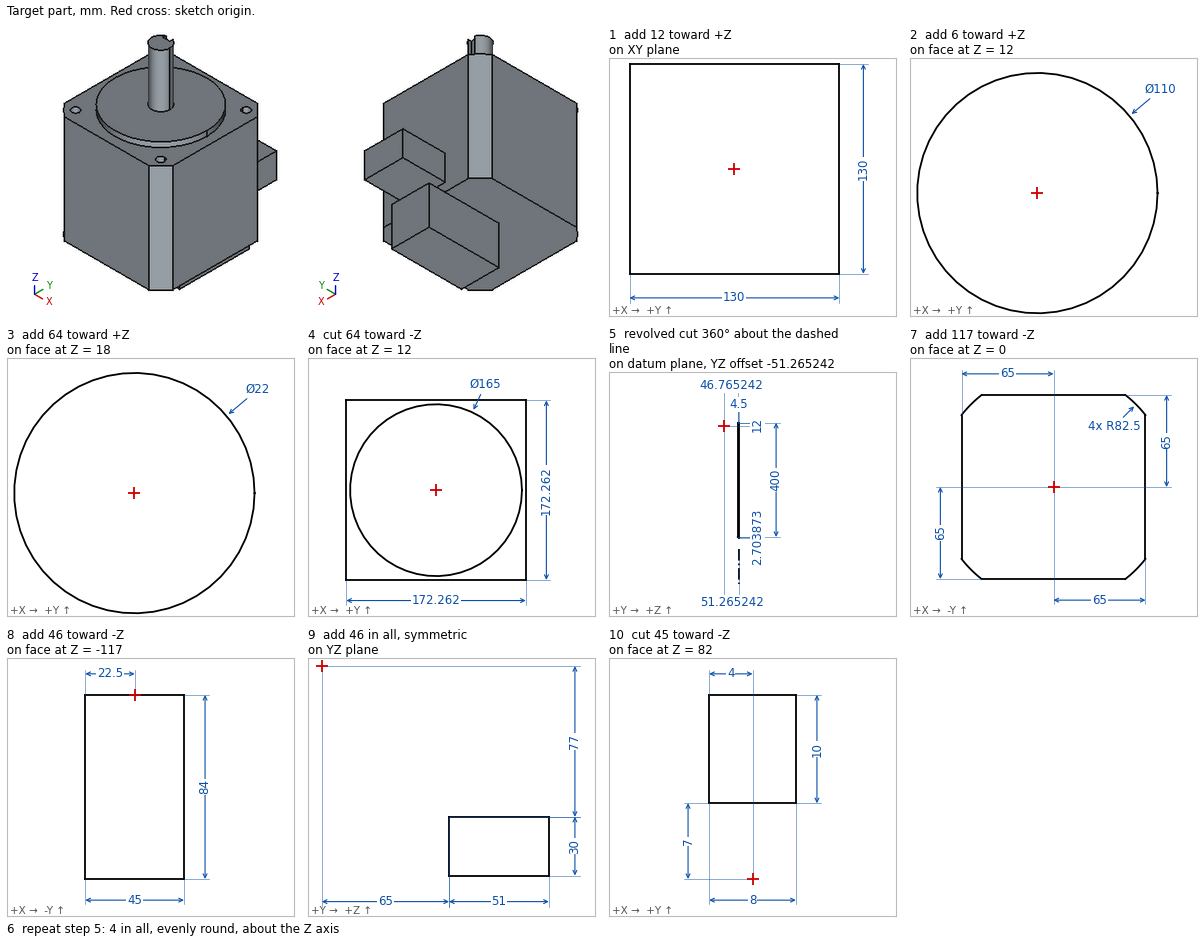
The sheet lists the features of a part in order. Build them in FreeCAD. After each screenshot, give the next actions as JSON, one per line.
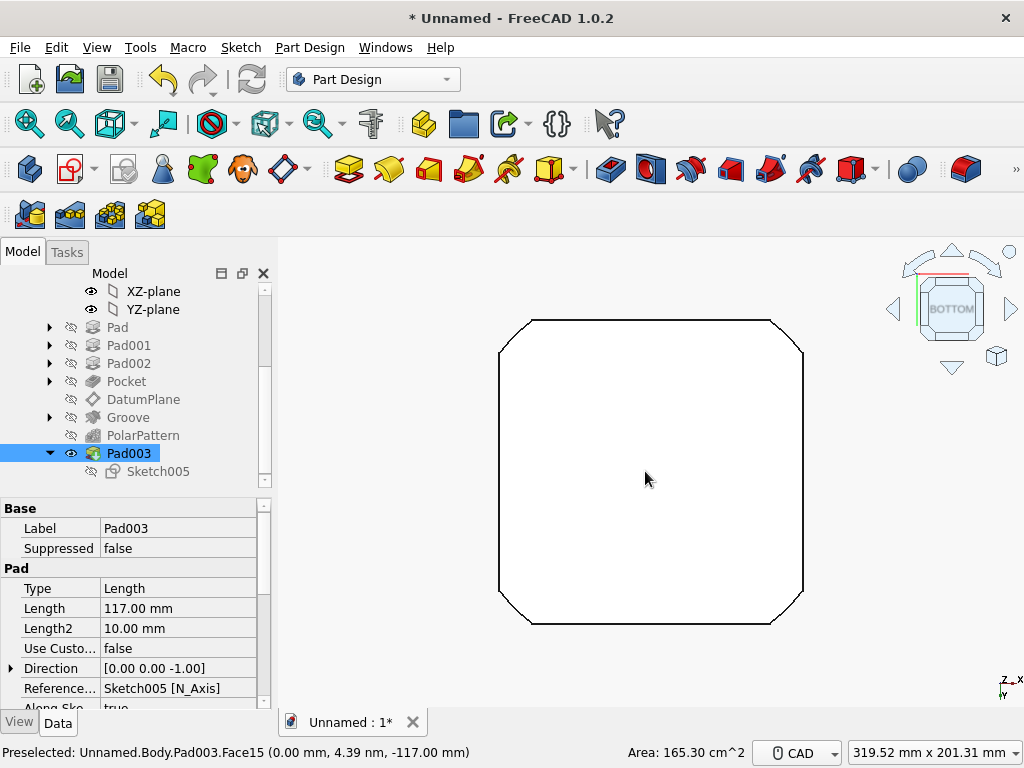
{"action": "left_click", "coordinate": [70, 170]}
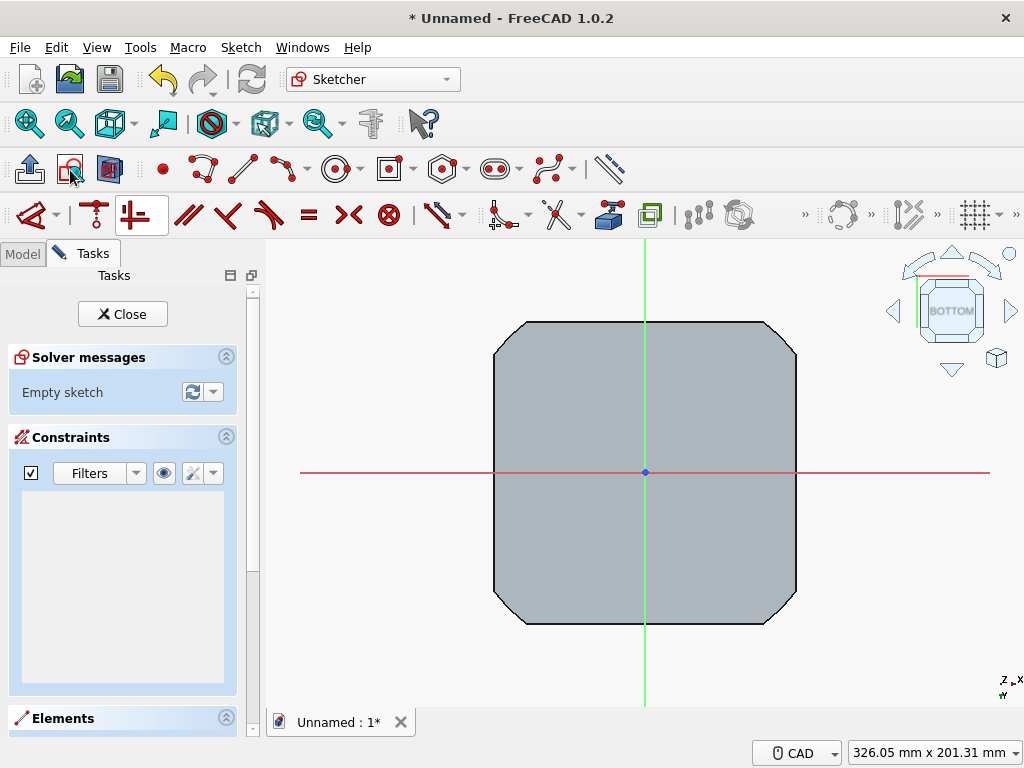
{"action": "scroll", "coordinate": [294, 267], "scroll_direction": "down", "scroll_amount": 1}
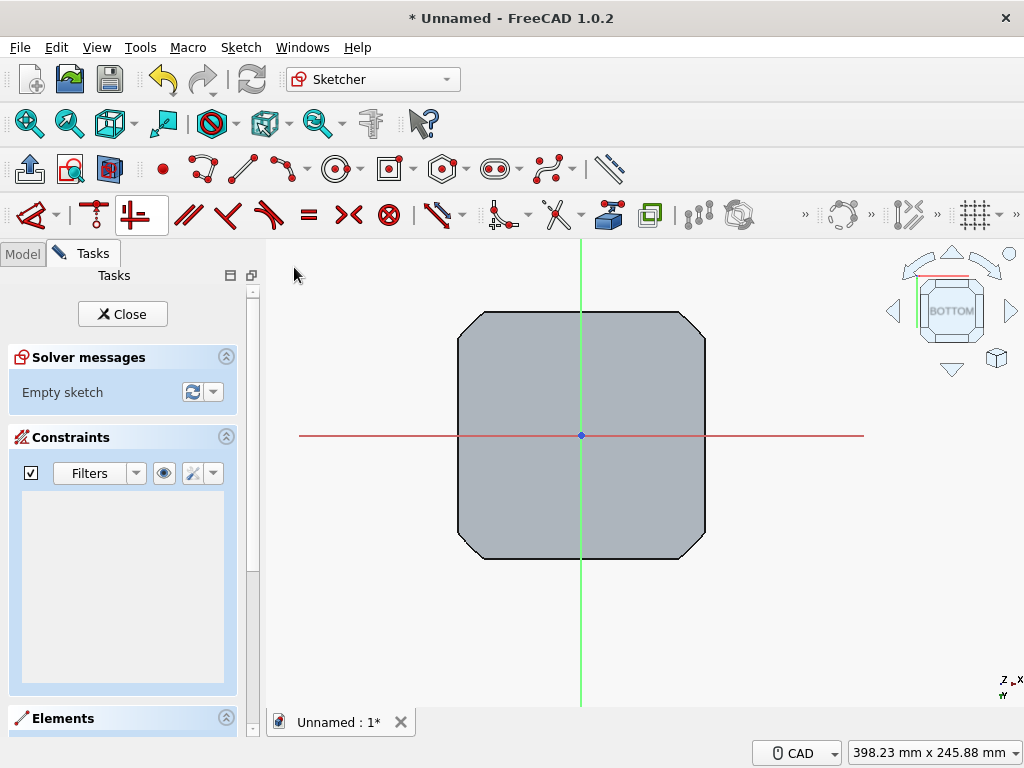
{"action": "scroll", "coordinate": [587, 567], "scroll_direction": "up", "scroll_amount": 3}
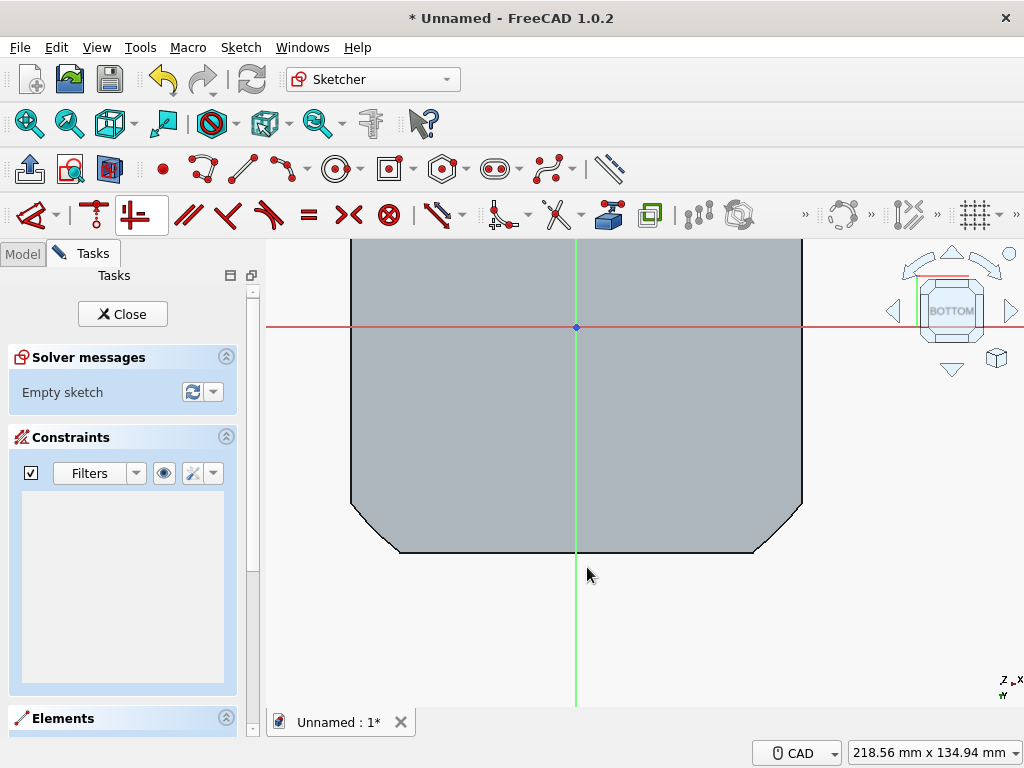
{"action": "key", "text": "g r"}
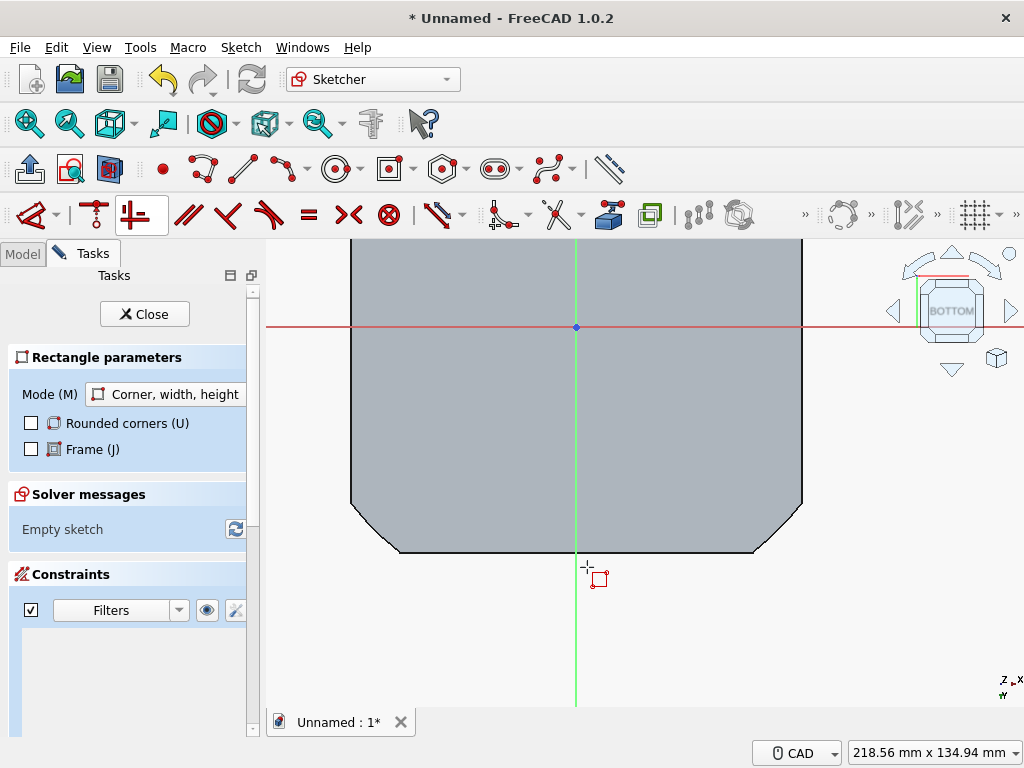
{"action": "left_click", "coordinate": [498, 327]}
{"action": "mouse_move", "coordinate": [654, 618]}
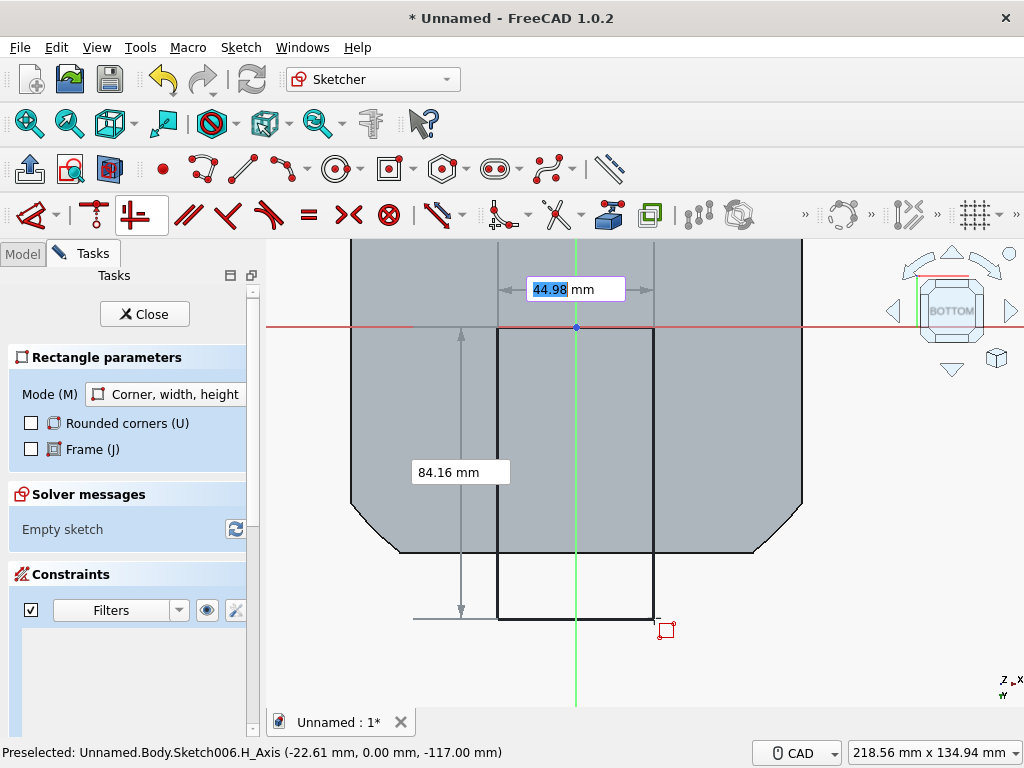
{"action": "type", "text": "45"}
{"action": "key", "text": "Tab"}
{"action": "type", "text": "84"}
{"action": "key", "text": "Return"}
{"action": "key", "text": "Escape"}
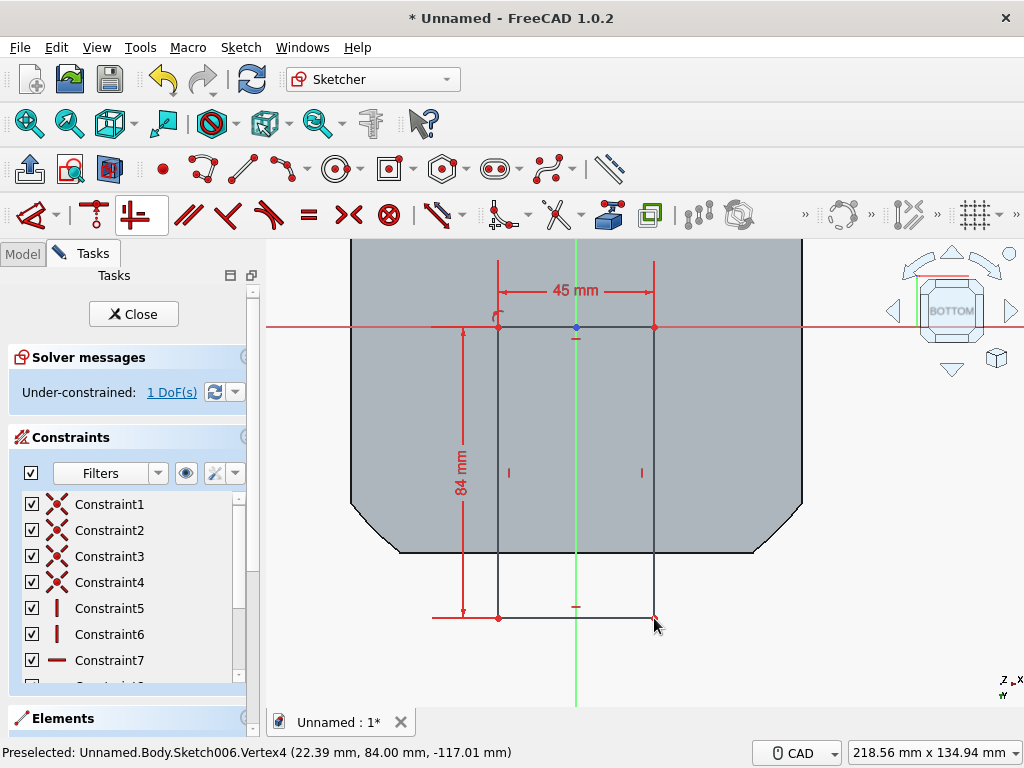
{"action": "left_click", "coordinate": [32, 216]}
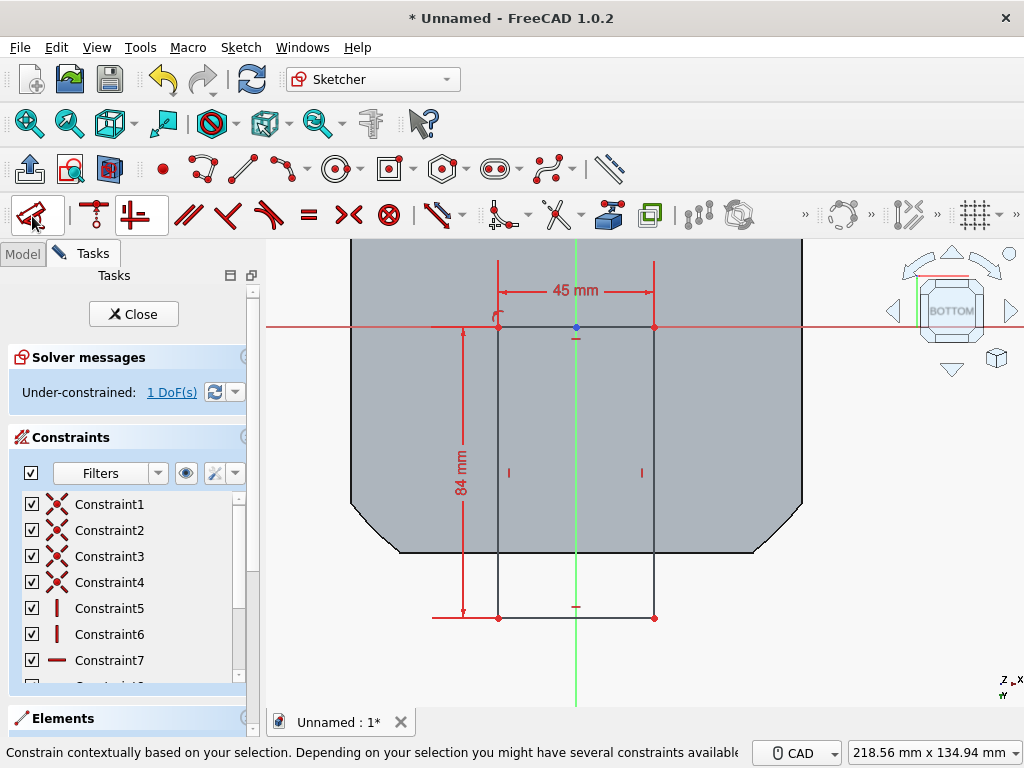
{"action": "left_click", "coordinate": [498, 327]}
{"action": "left_click", "coordinate": [537, 293]}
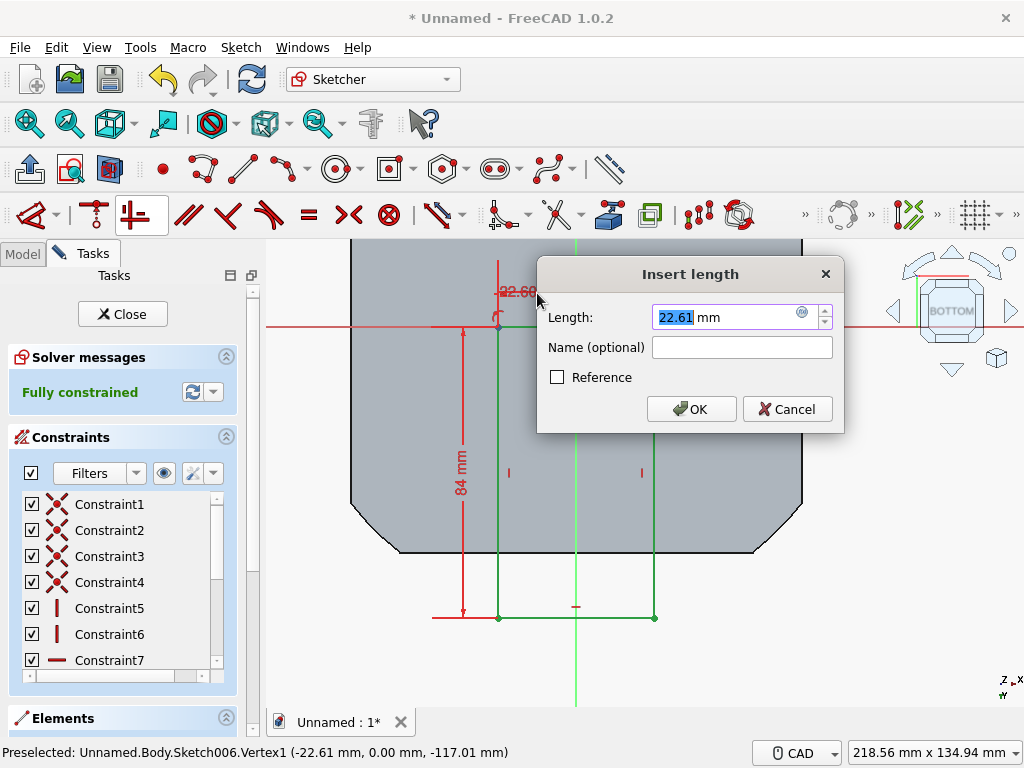
{"action": "type", "text": "22.5"}
{"action": "key", "text": "Return"}
{"action": "key", "text": "Escape"}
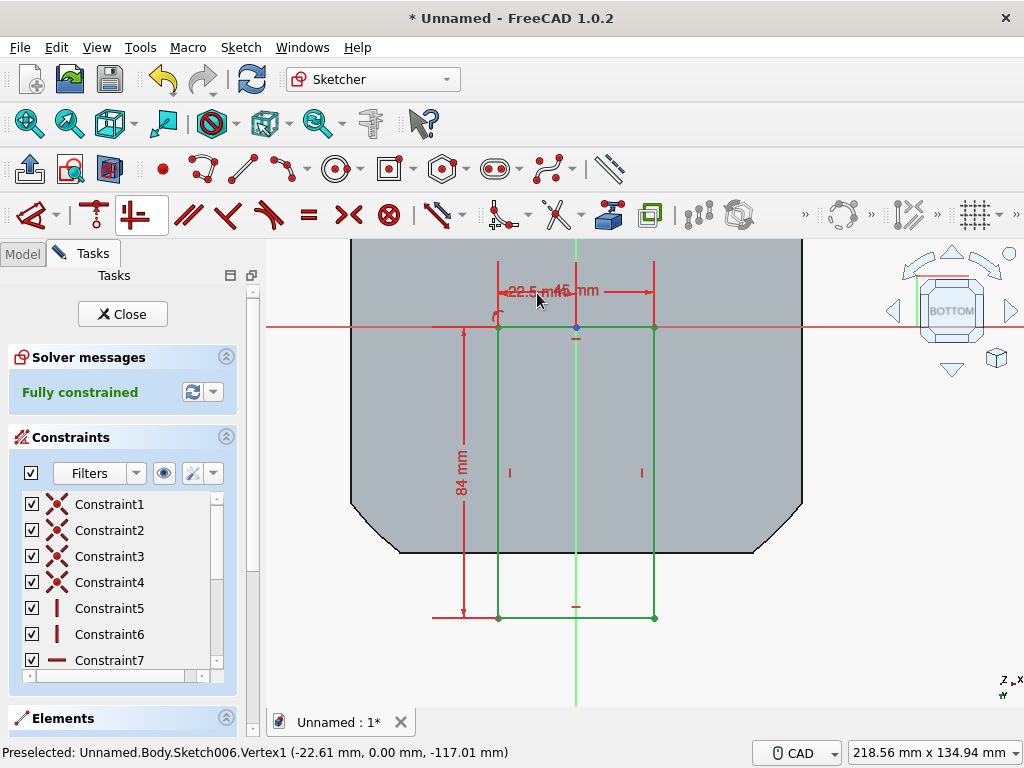
{"action": "left_click", "coordinate": [123, 314]}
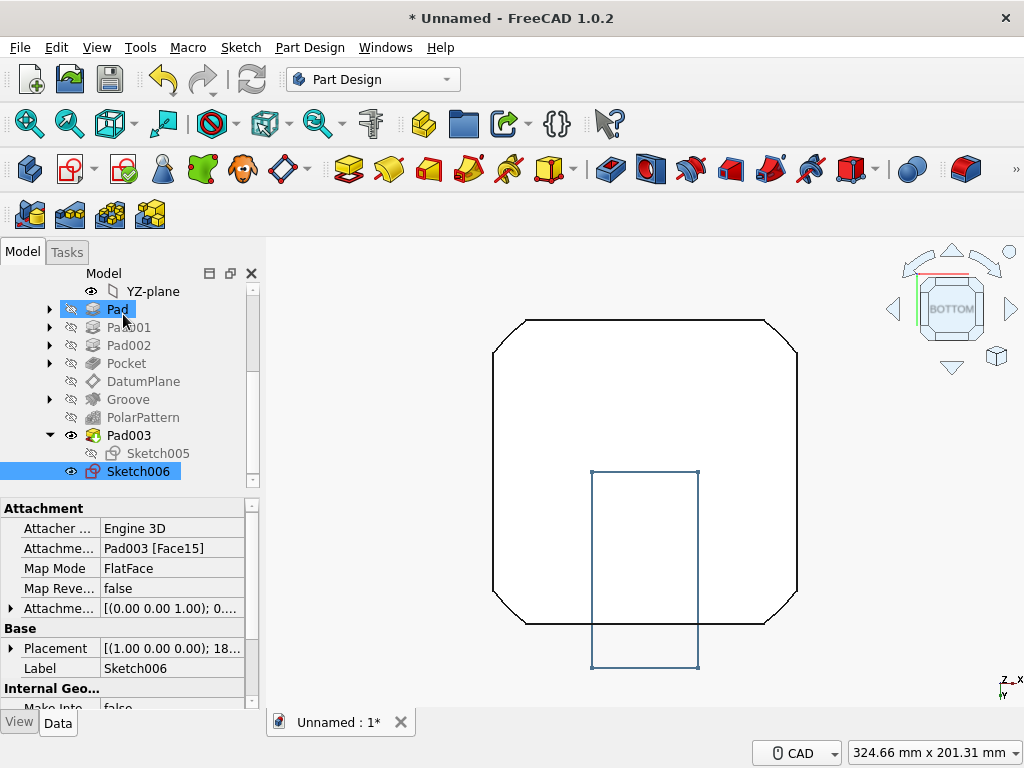
{"action": "left_click", "coordinate": [350, 170]}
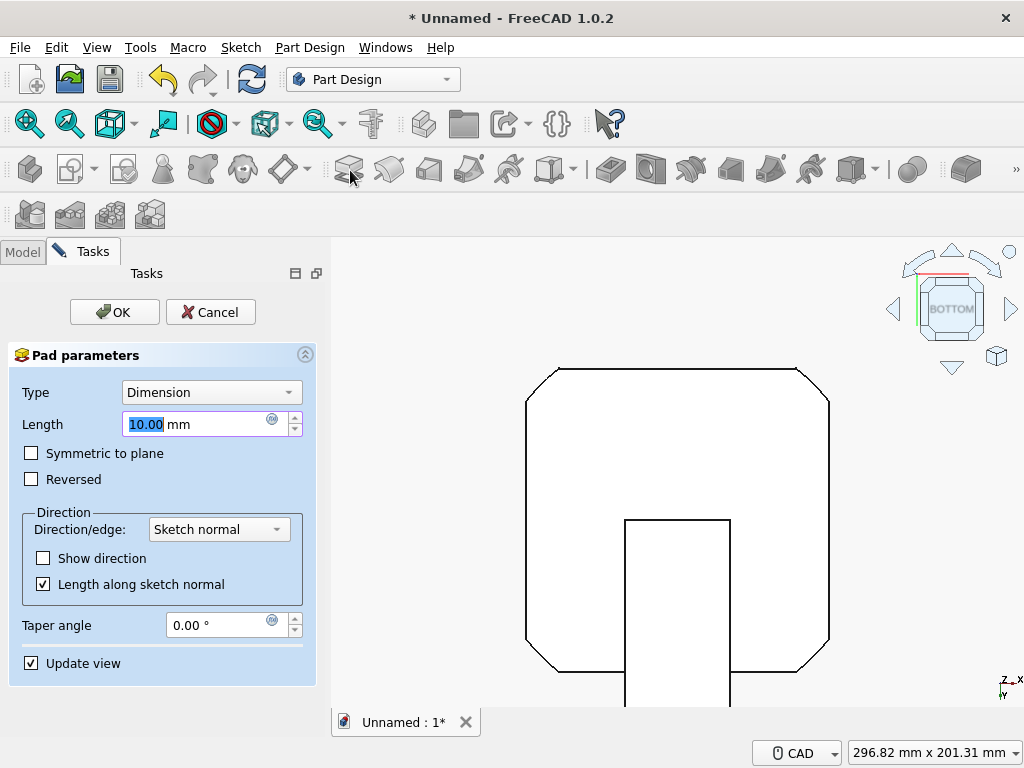
{"action": "type", "text": "46"}
{"action": "key", "text": "Tab"}